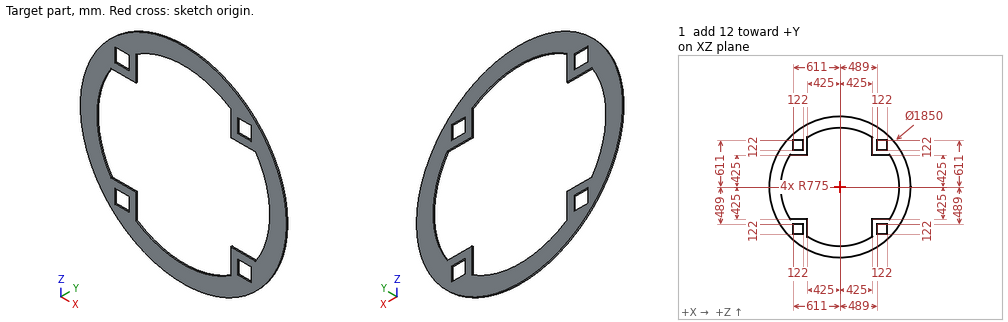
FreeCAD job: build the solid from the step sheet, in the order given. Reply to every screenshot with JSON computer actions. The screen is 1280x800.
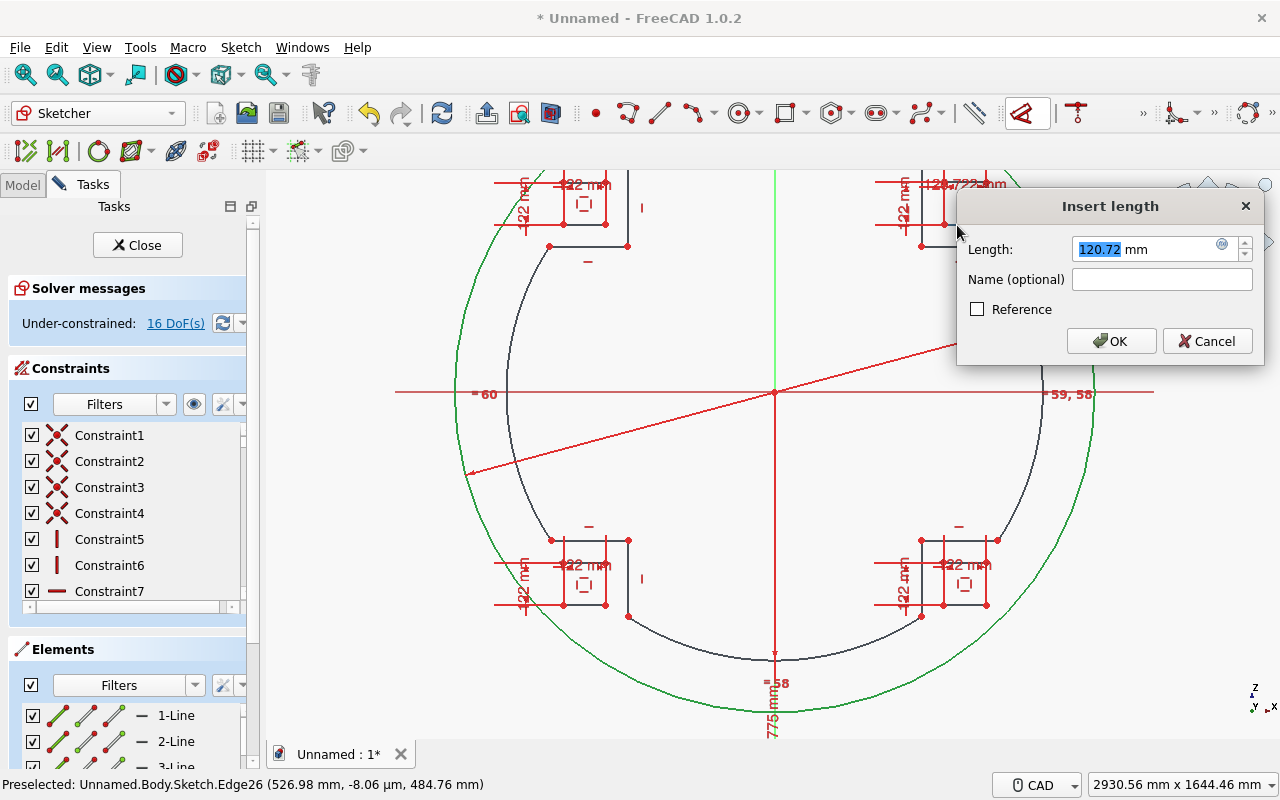
{"action": "type", "text": "122"}
{"action": "key", "text": "Return"}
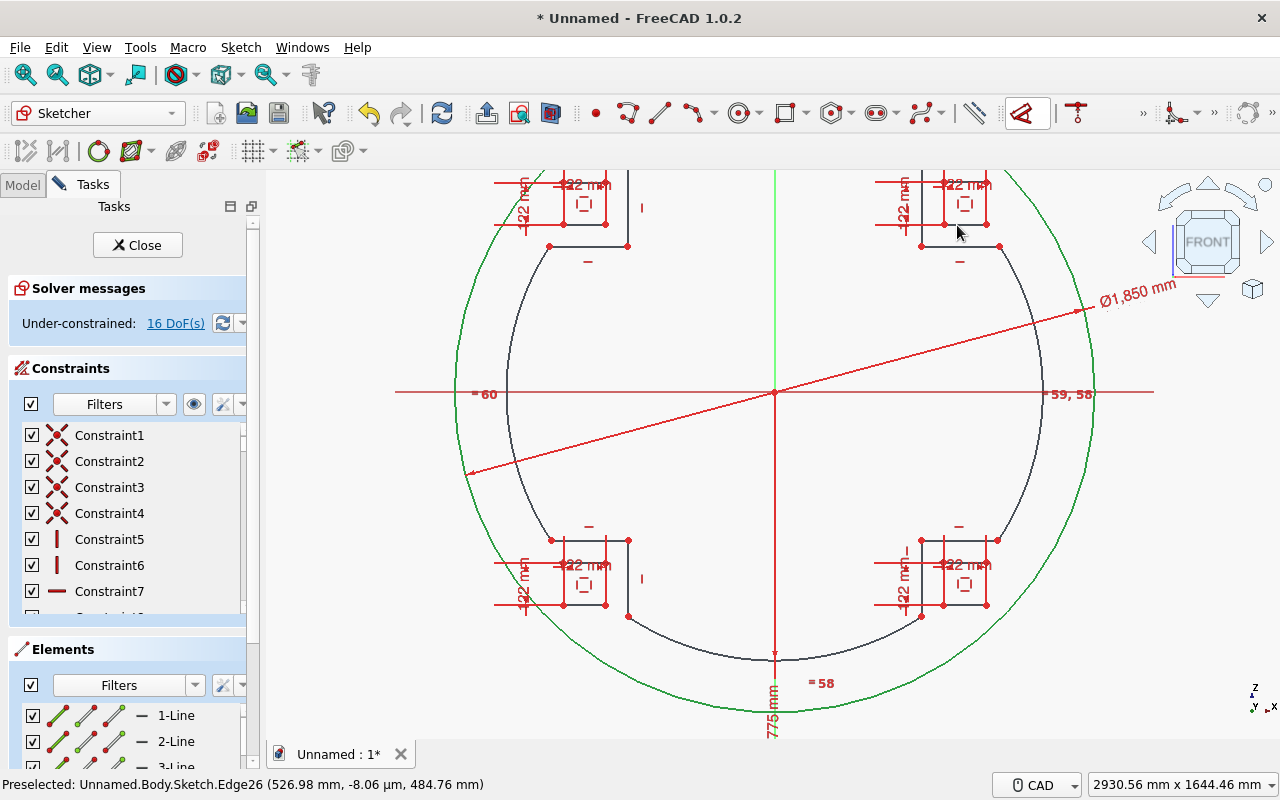
{"action": "left_click", "coordinate": [564, 563]}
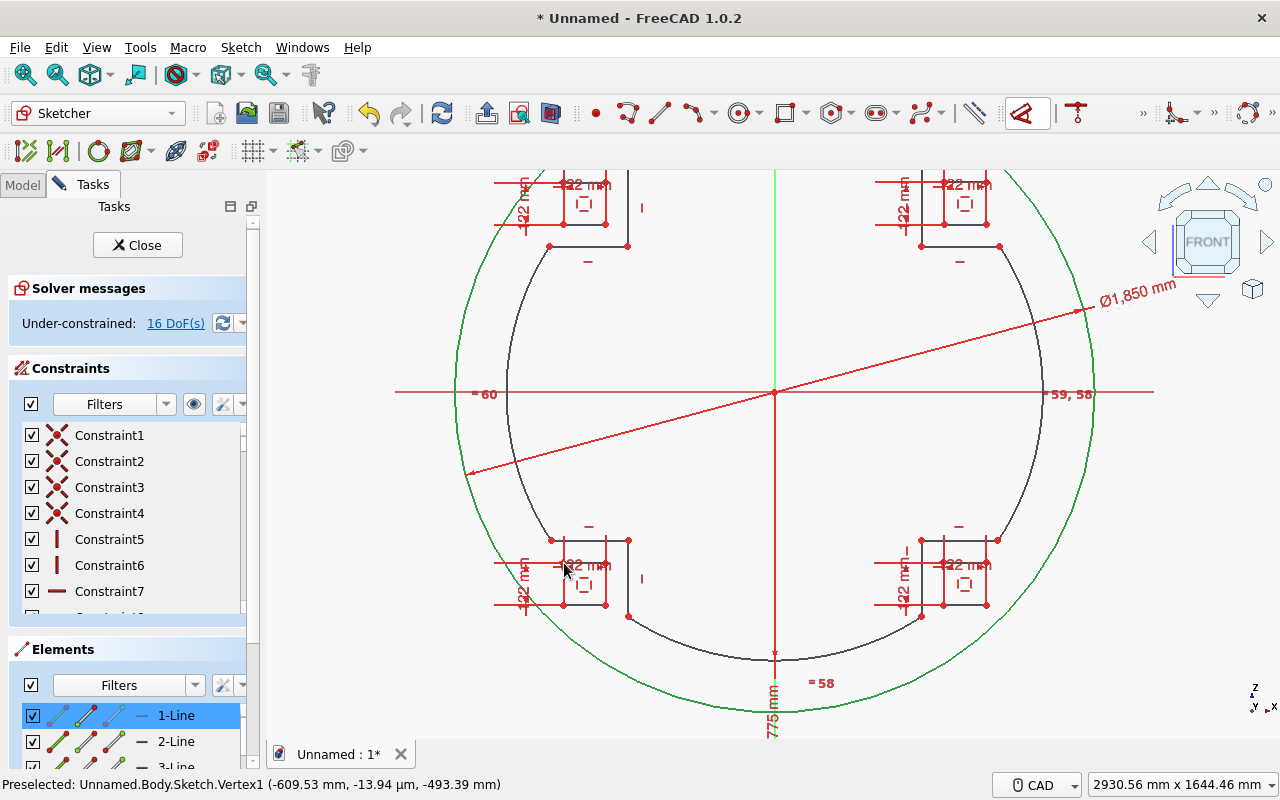
{"action": "key", "text": "l"}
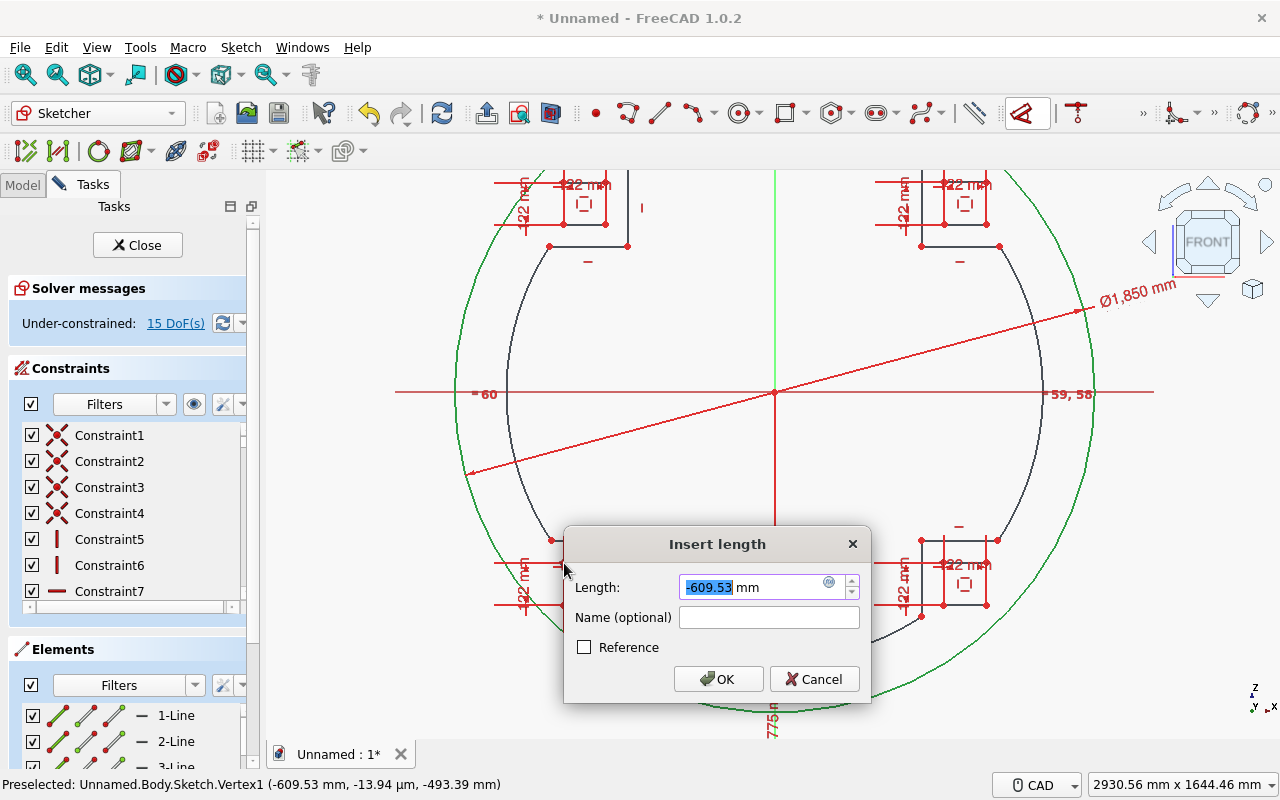
{"action": "type", "text": "-611"}
{"action": "key", "text": "Return"}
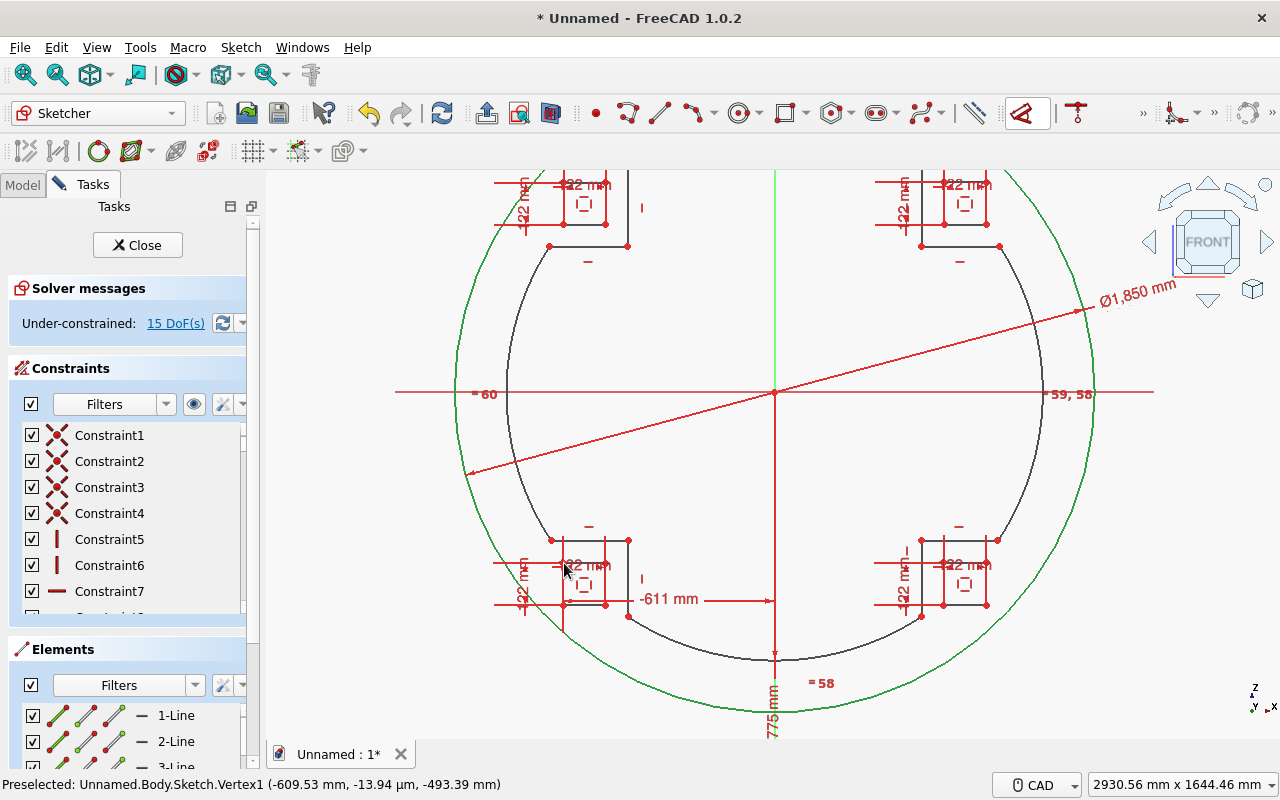
{"action": "left_click", "coordinate": [563, 563]}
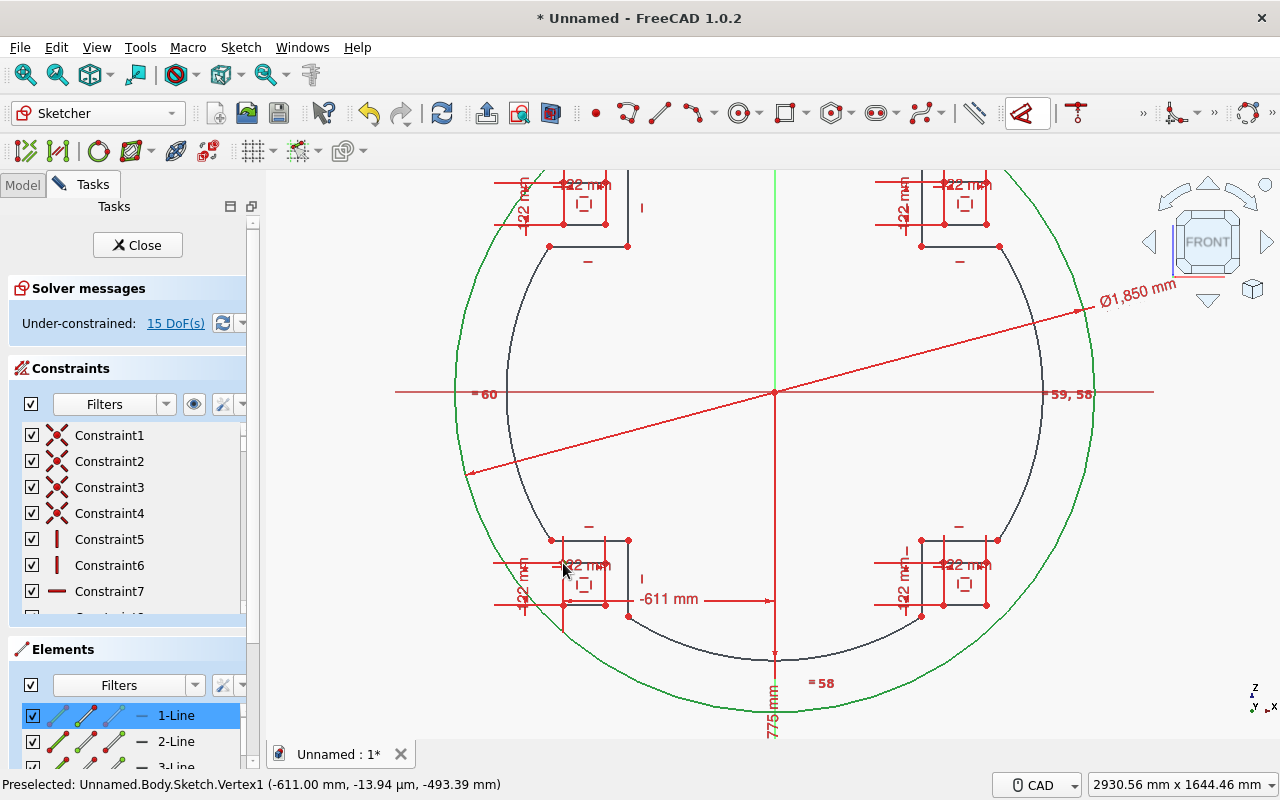
{"action": "key", "text": "i"}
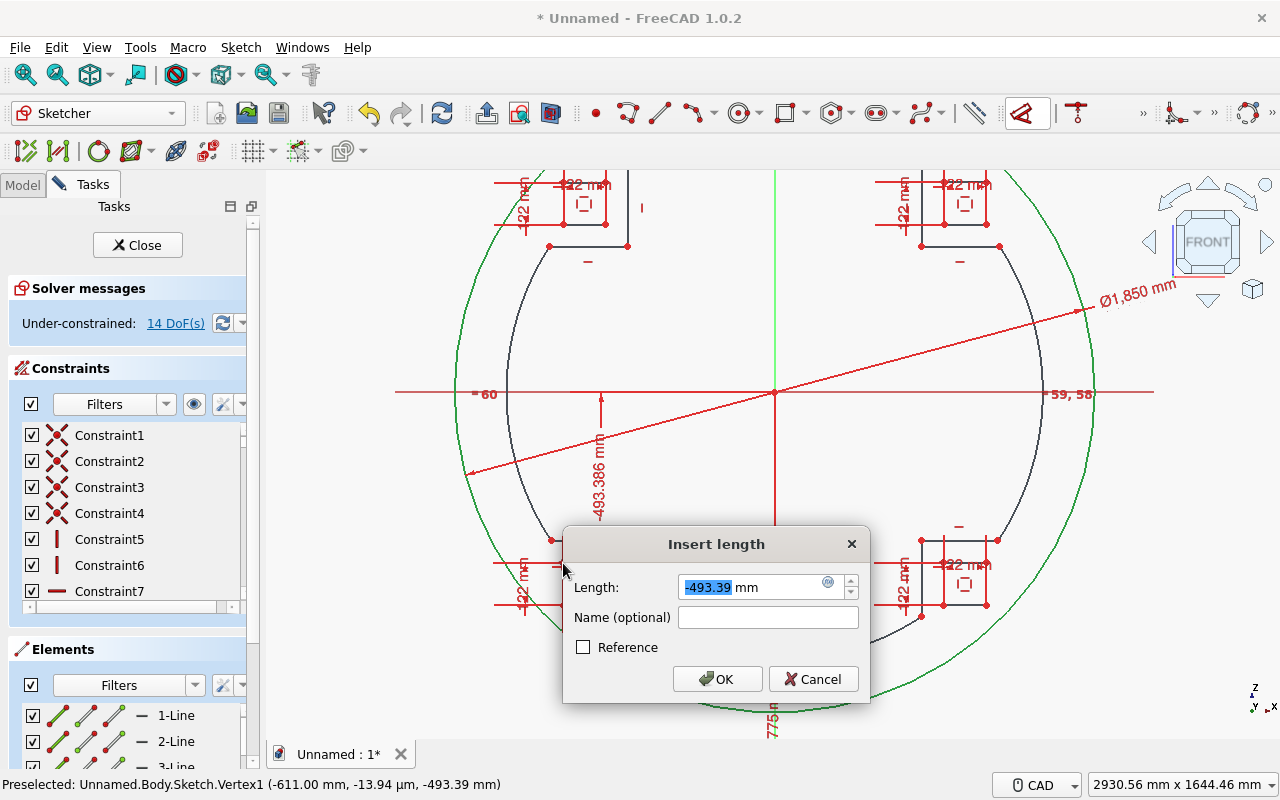
{"action": "type", "text": "-489"}
{"action": "key", "text": "Return"}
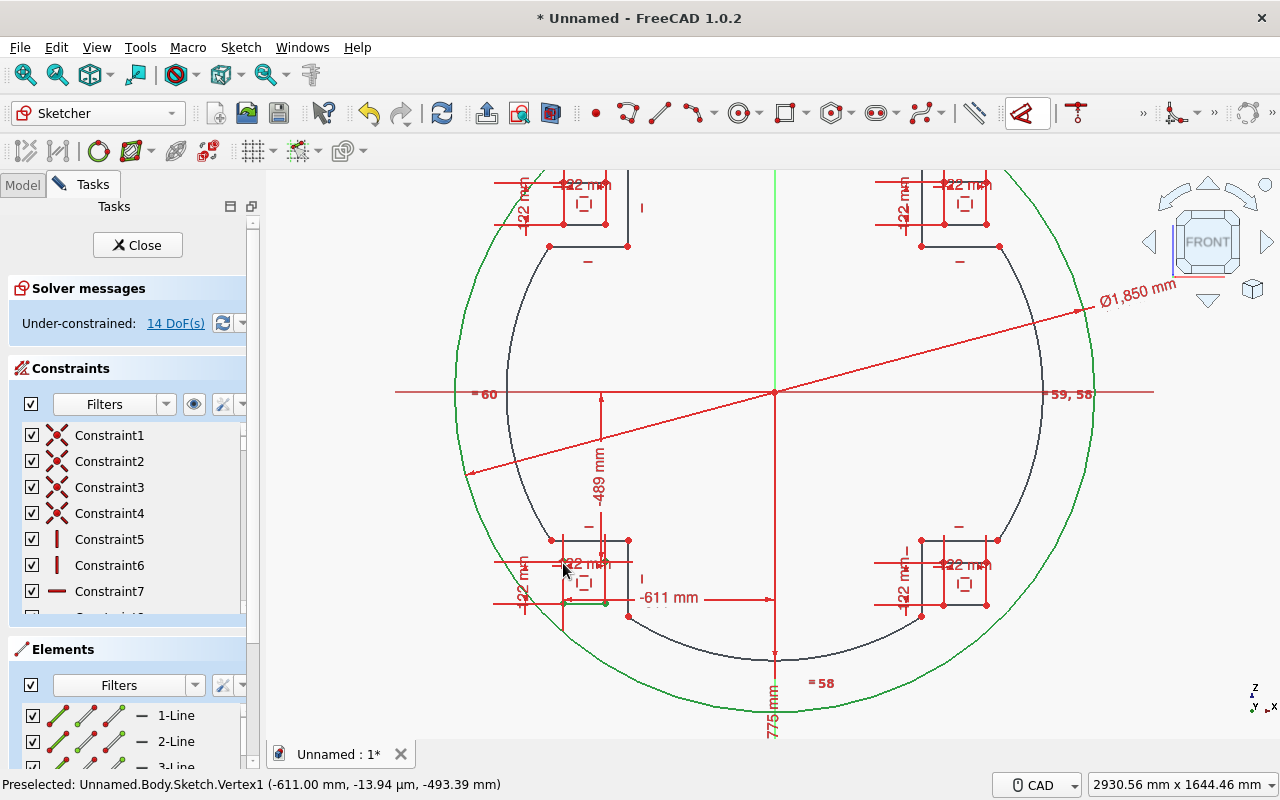
{"action": "scroll", "coordinate": [619, 530], "scroll_direction": "down", "scroll_amount": 3}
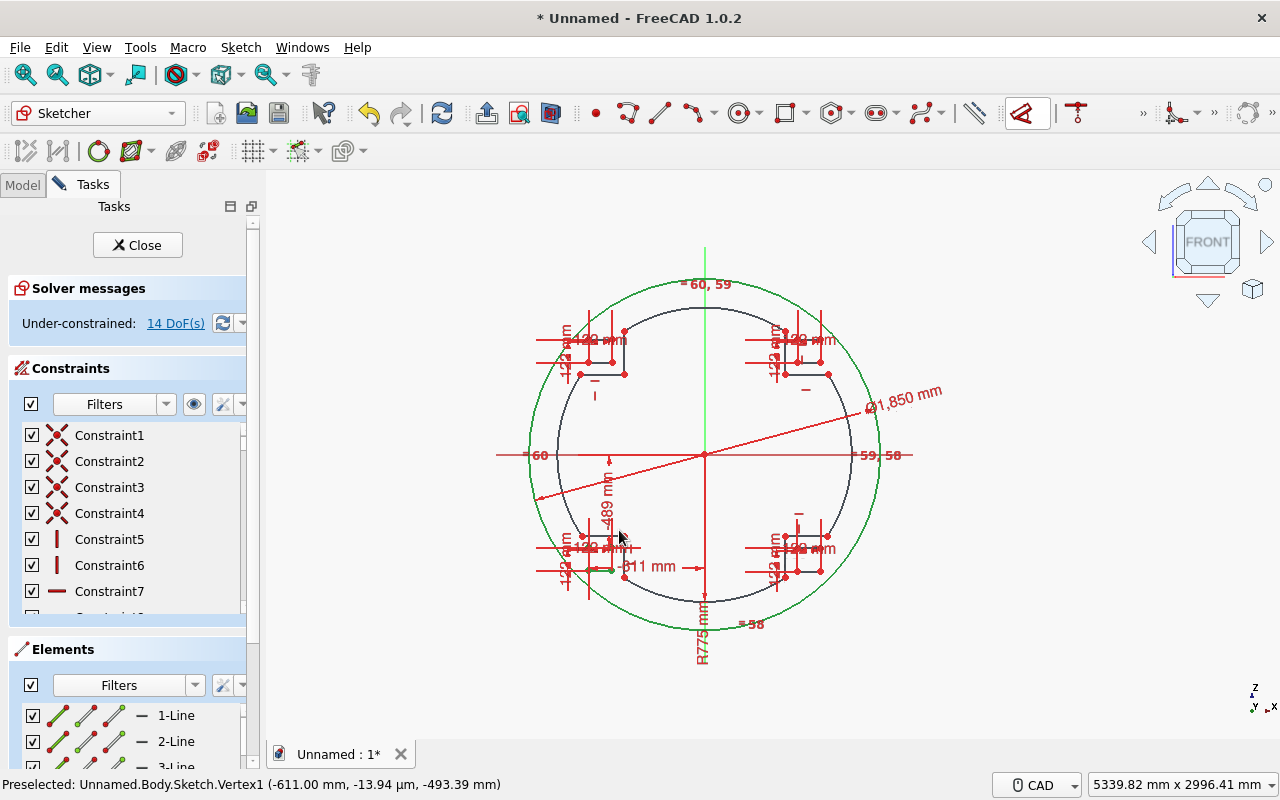
{"action": "left_click", "coordinate": [589, 340]}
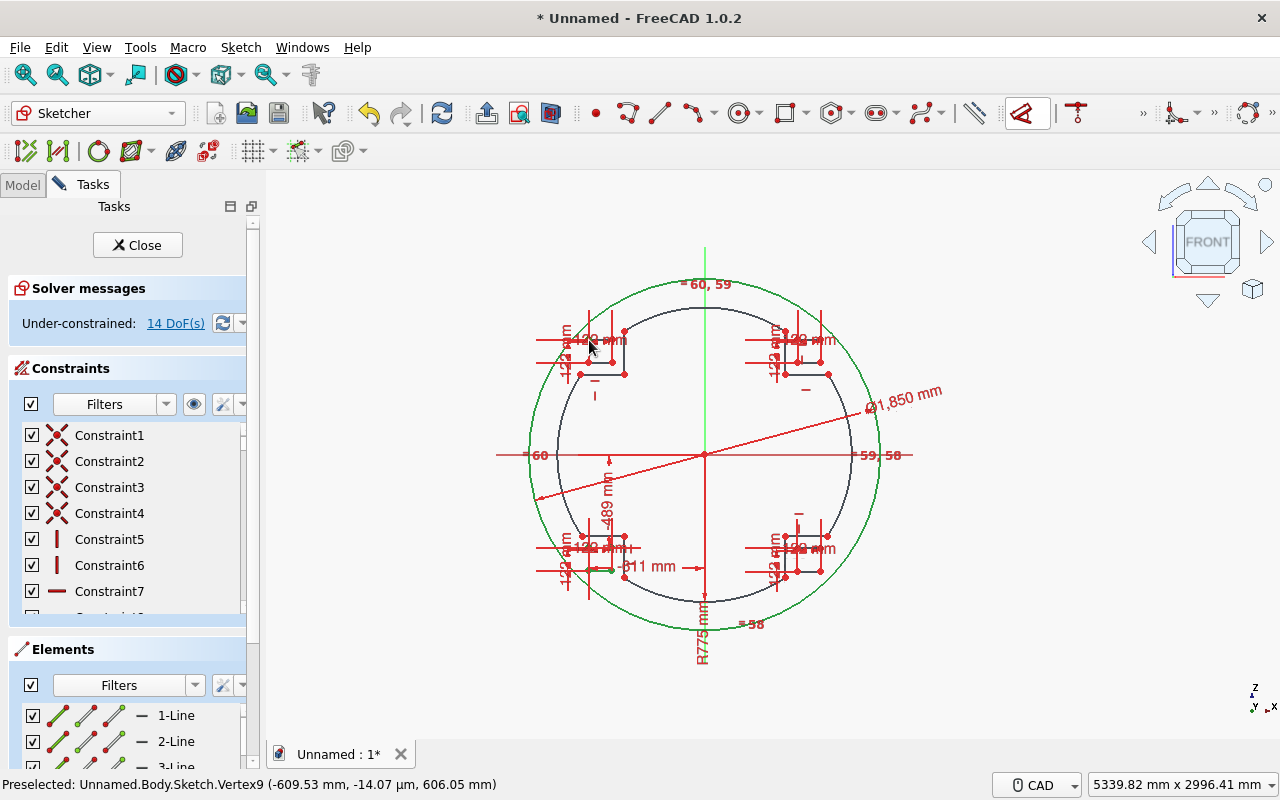
{"action": "key", "text": "l"}